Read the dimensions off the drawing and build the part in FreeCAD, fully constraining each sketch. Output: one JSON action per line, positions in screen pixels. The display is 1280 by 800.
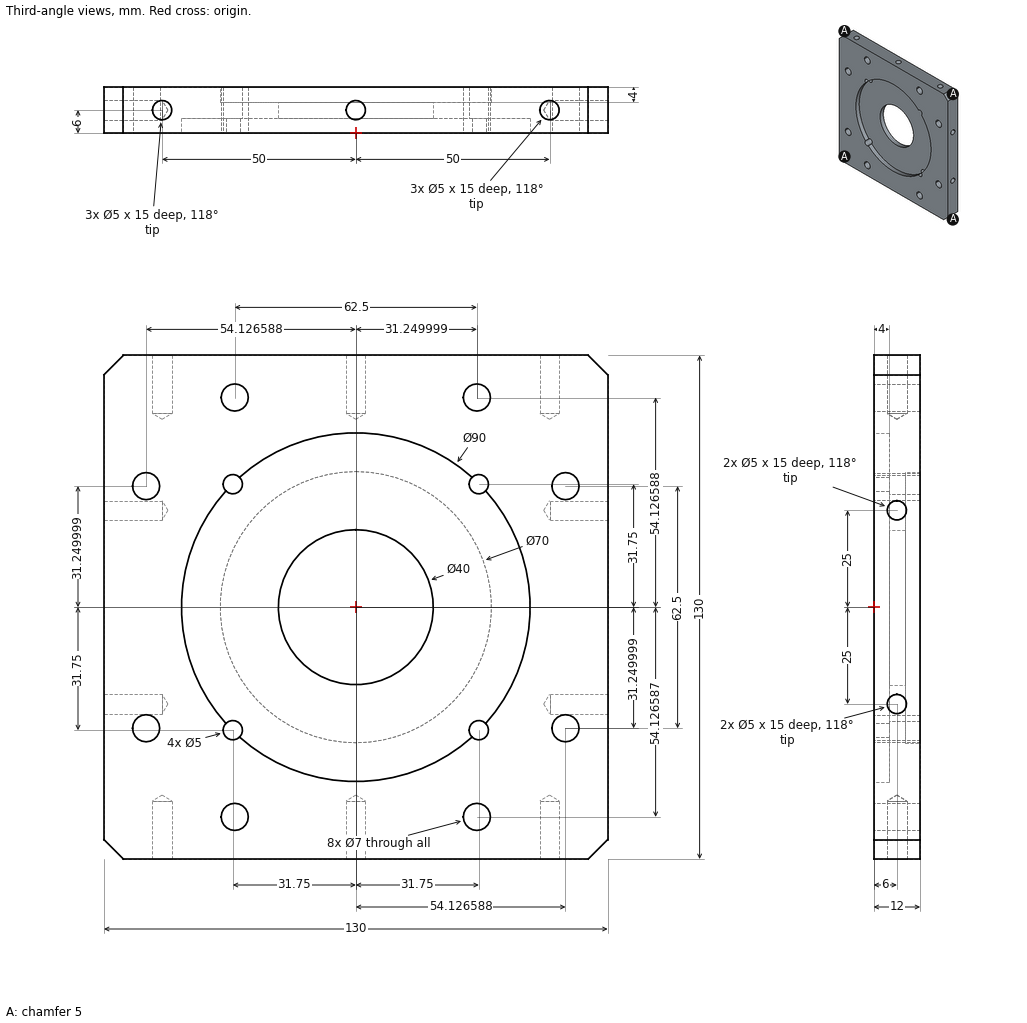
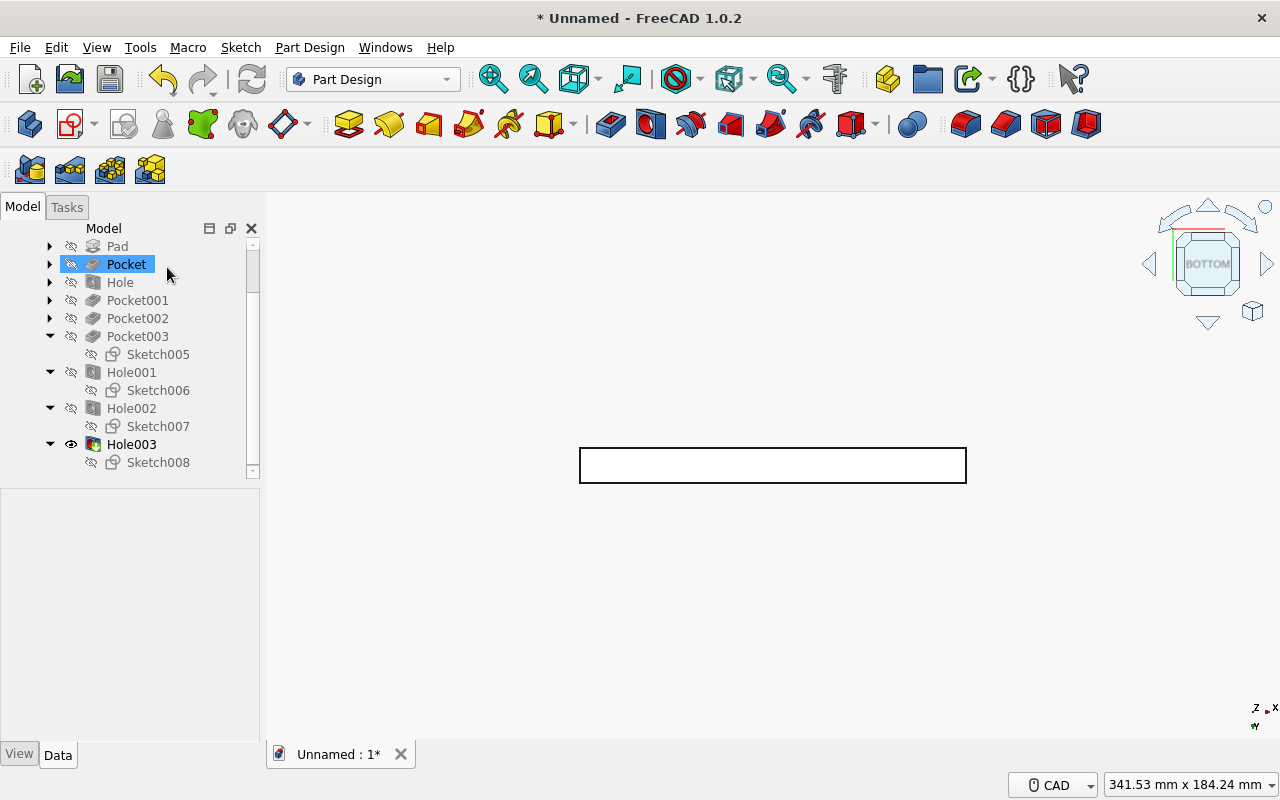
{"action": "key", "text": "v f"}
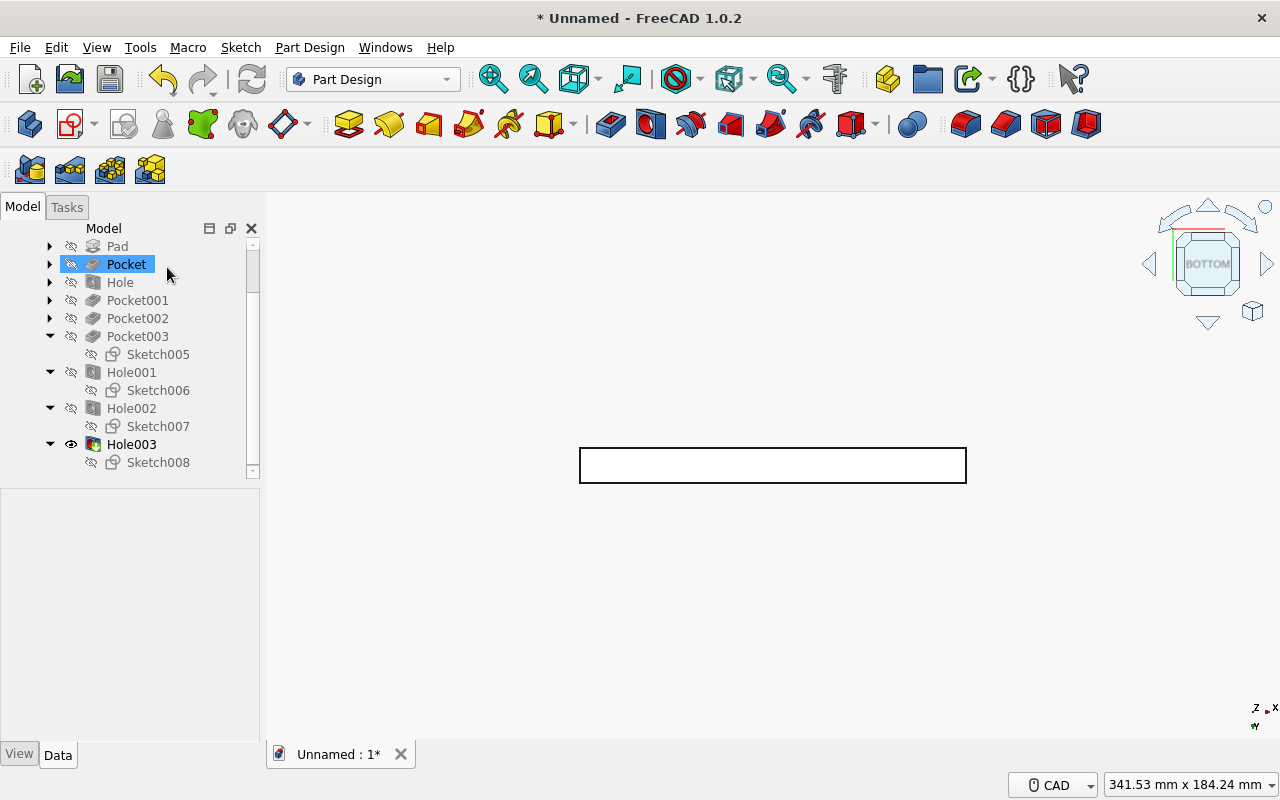
{"action": "left_click", "coordinate": [938, 464]}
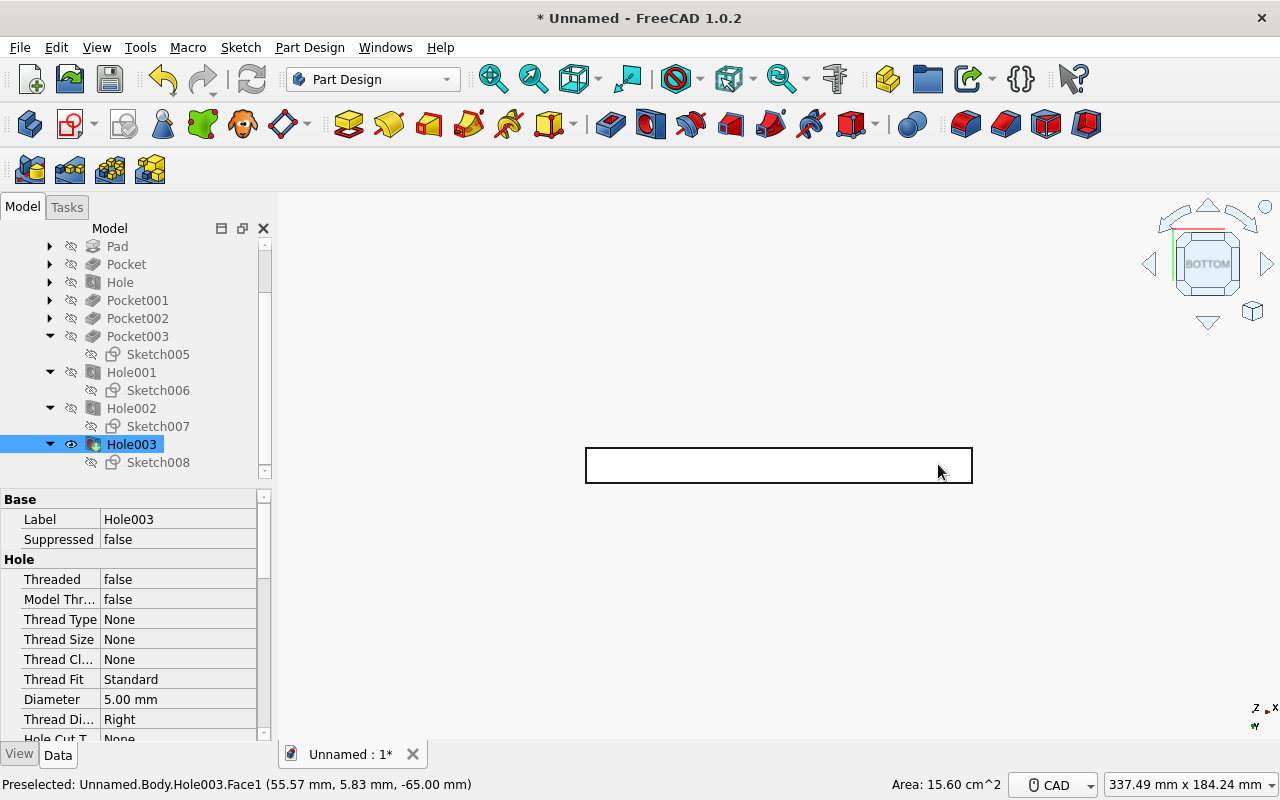
{"action": "left_click", "coordinate": [70, 124]}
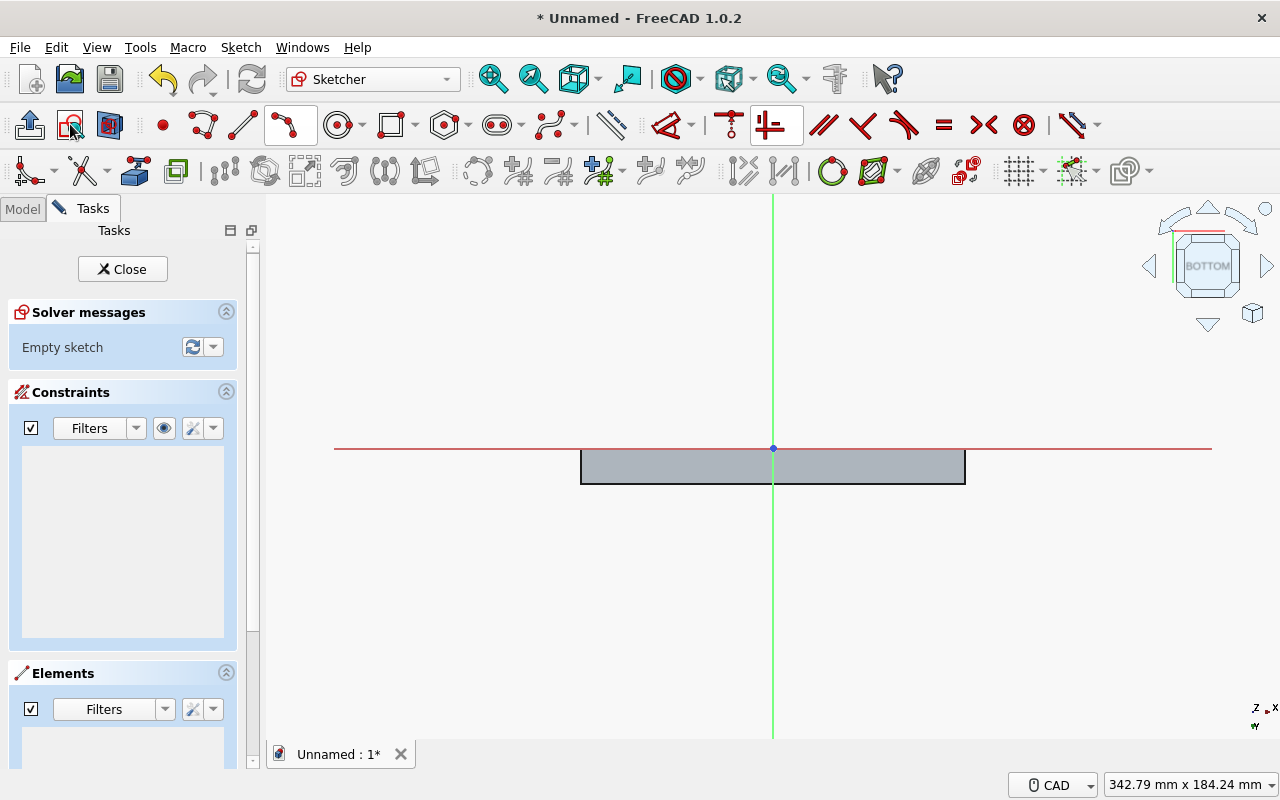
{"action": "scroll", "coordinate": [856, 455], "scroll_direction": "up", "scroll_amount": 3}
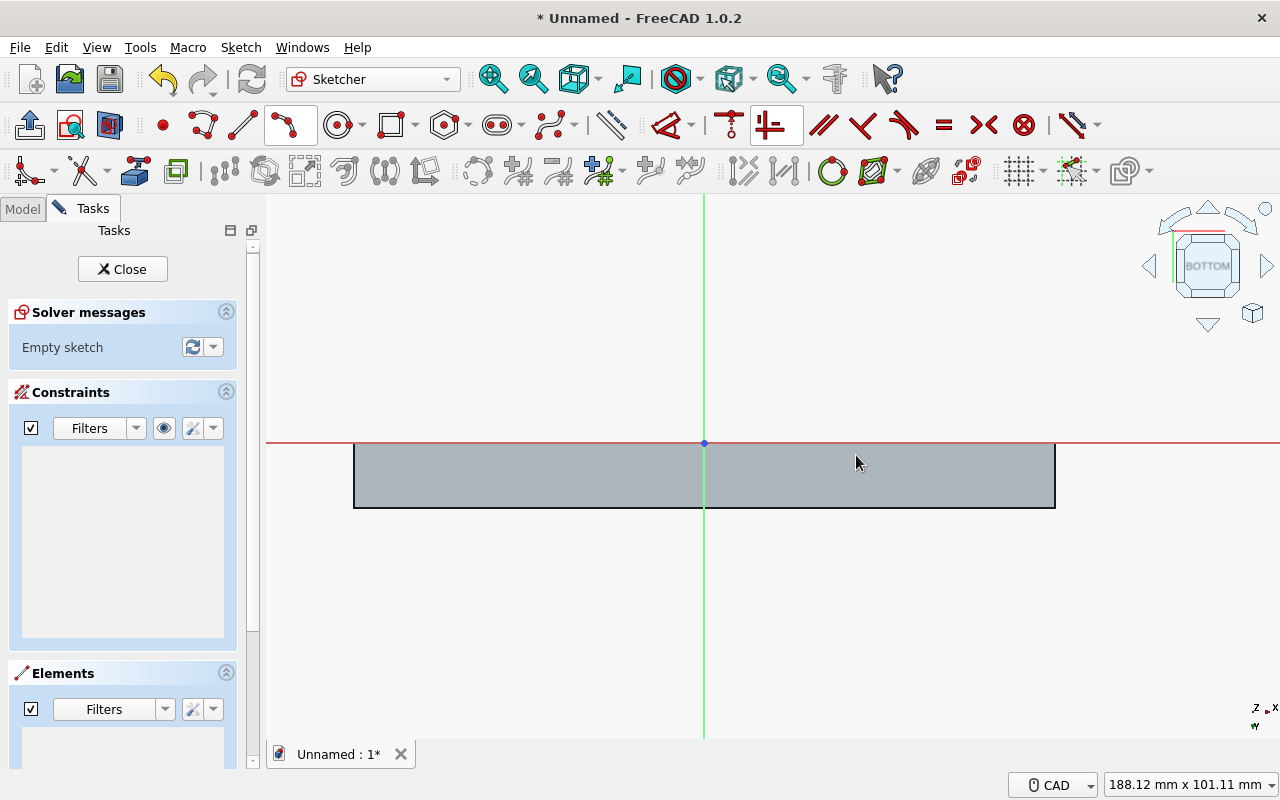
{"action": "key", "text": "g c"}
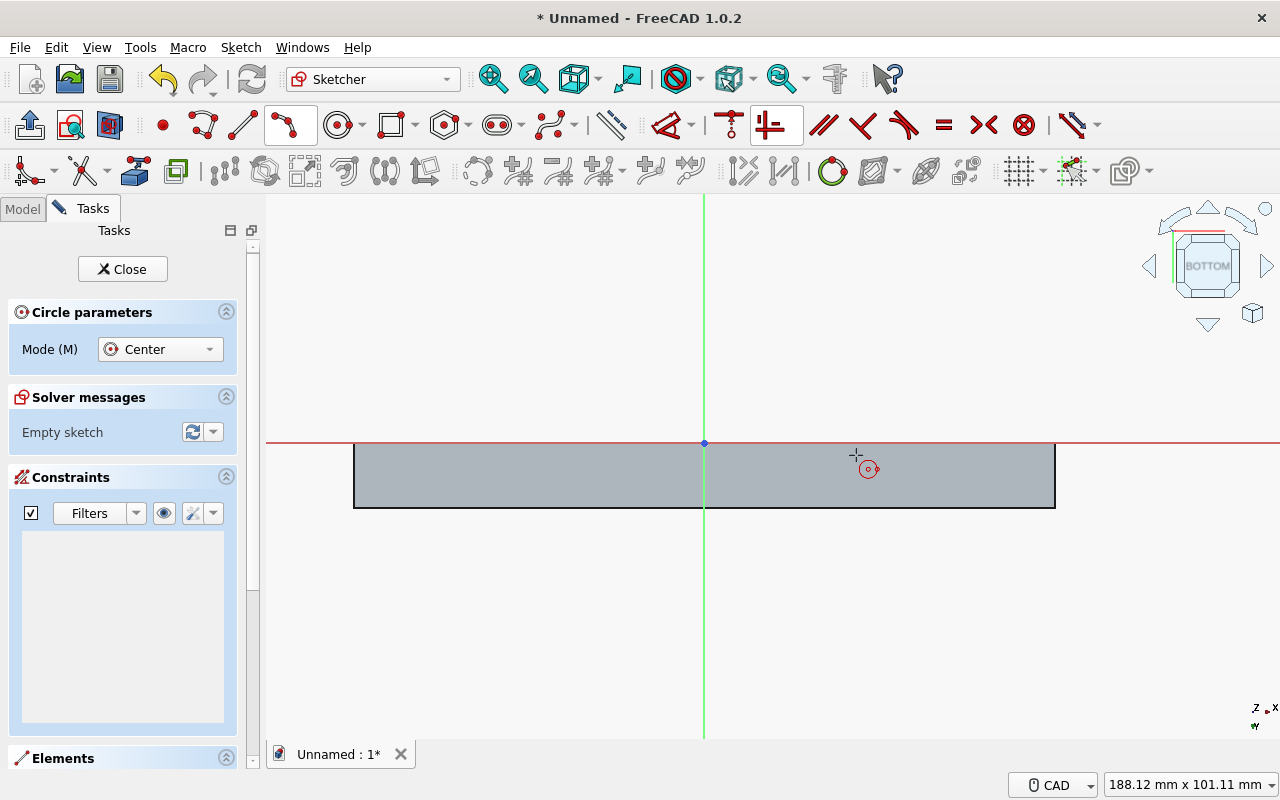
{"action": "scroll", "coordinate": [974, 476], "scroll_direction": "up", "scroll_amount": 3}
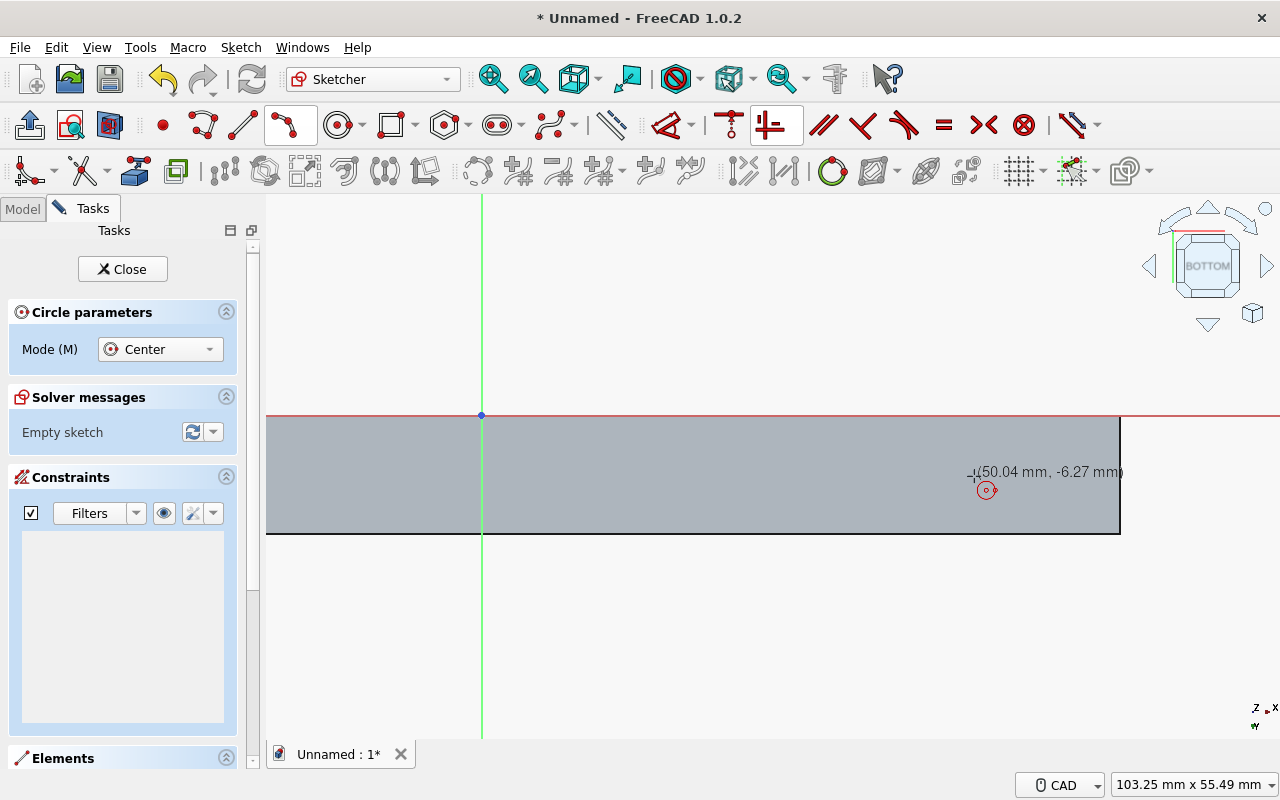
{"action": "left_click", "coordinate": [973, 475]}
{"action": "left_click", "coordinate": [990, 457]}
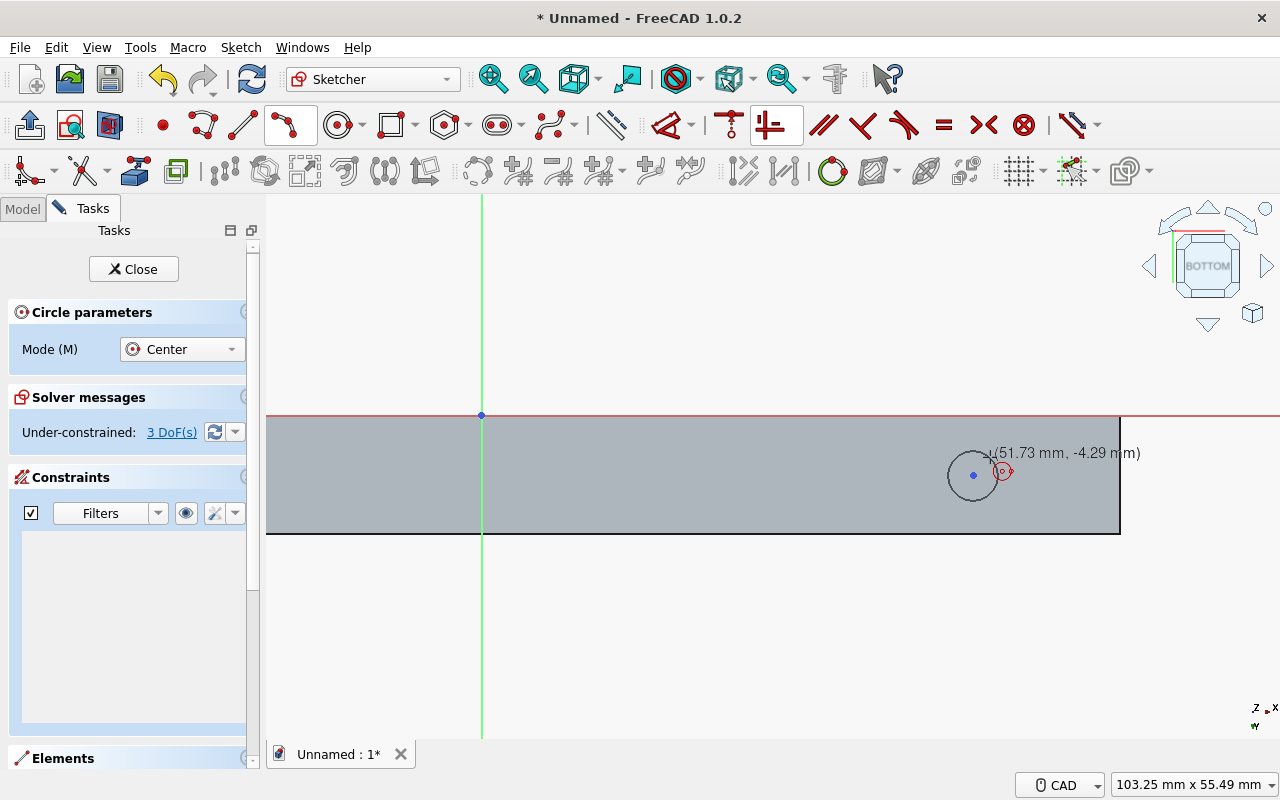
{"action": "scroll", "coordinate": [975, 477], "scroll_direction": "down", "scroll_amount": 3}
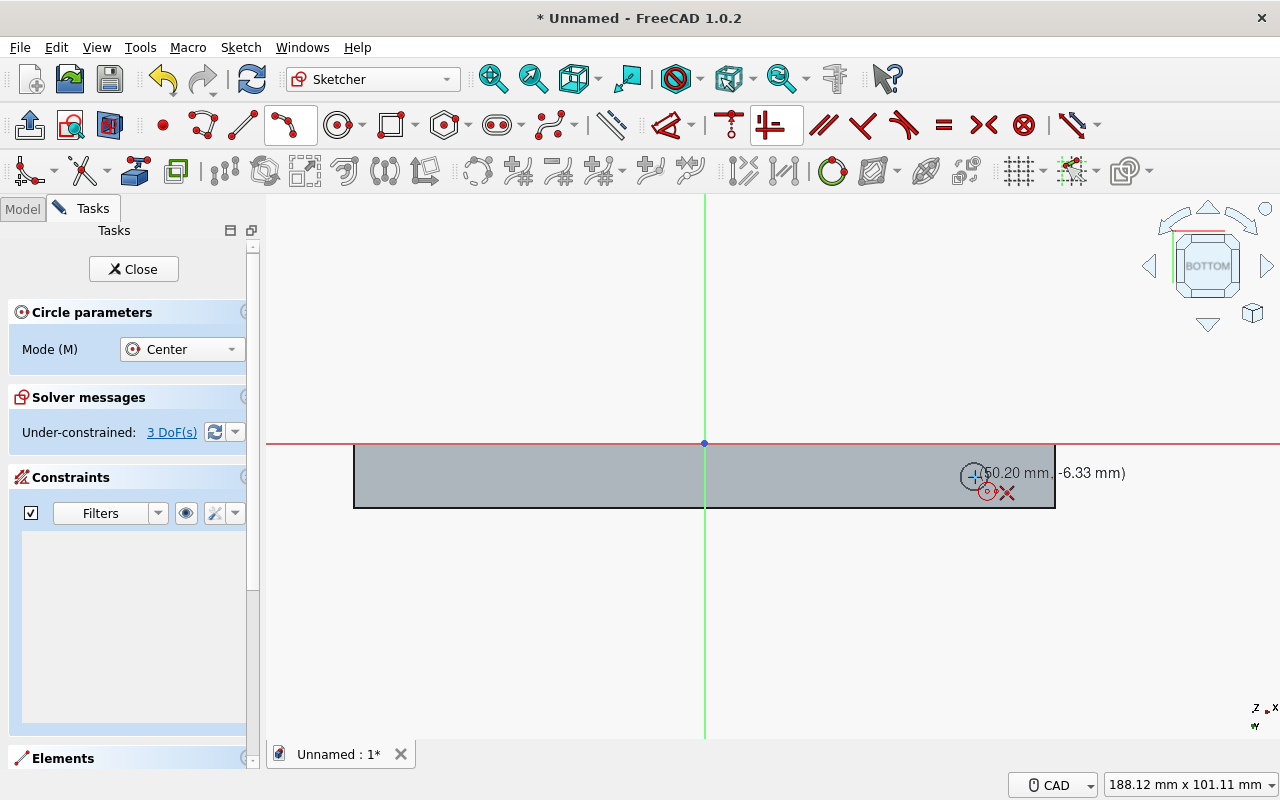
{"action": "scroll", "coordinate": [435, 476], "scroll_direction": "up", "scroll_amount": 3}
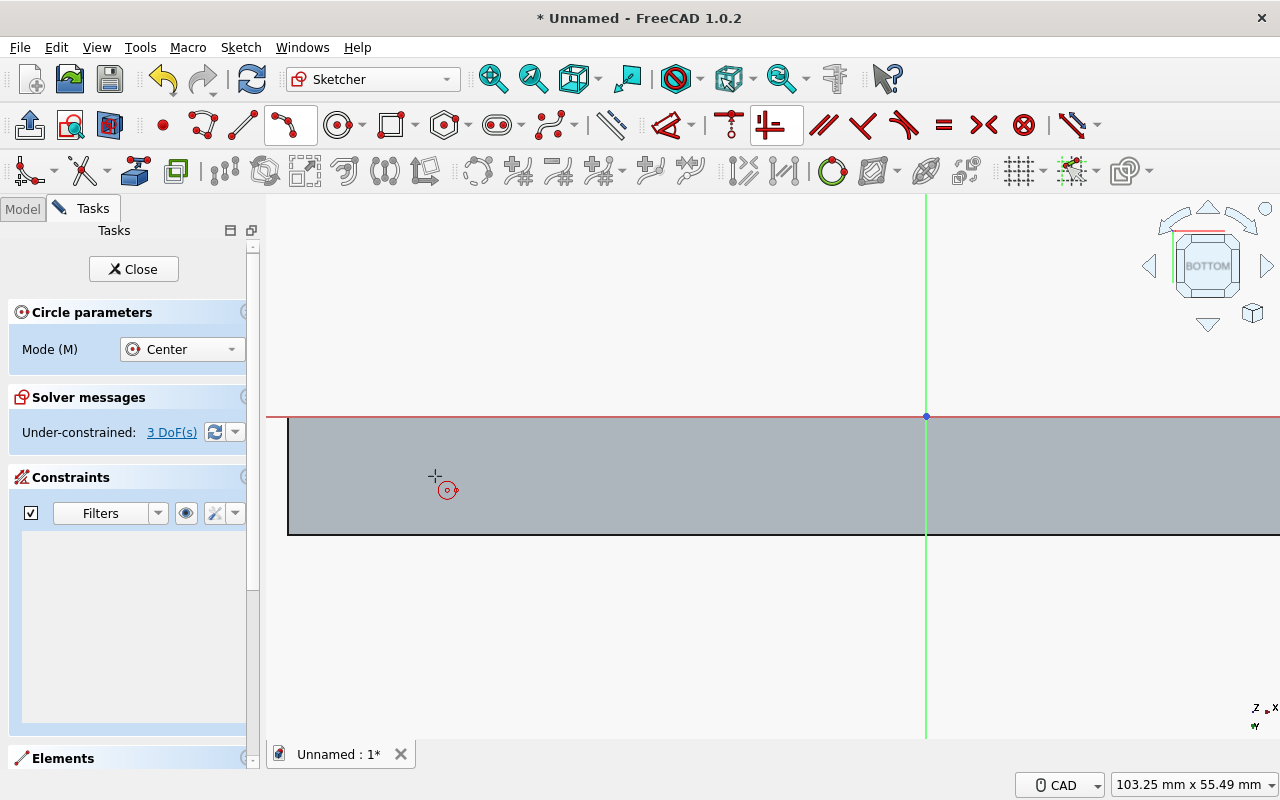
{"action": "left_click", "coordinate": [435, 476]}
{"action": "left_click", "coordinate": [453, 458]}